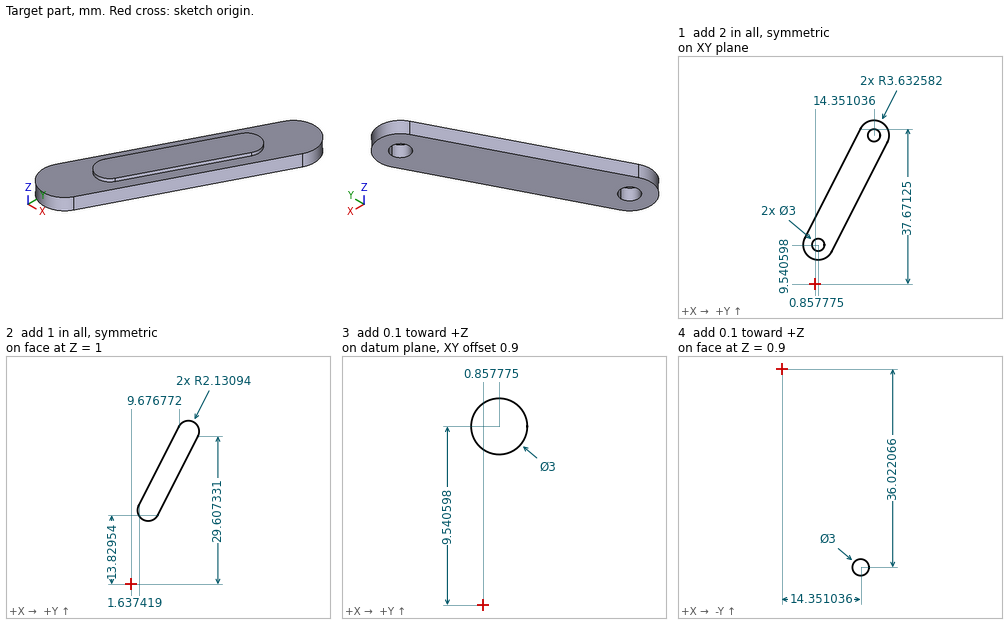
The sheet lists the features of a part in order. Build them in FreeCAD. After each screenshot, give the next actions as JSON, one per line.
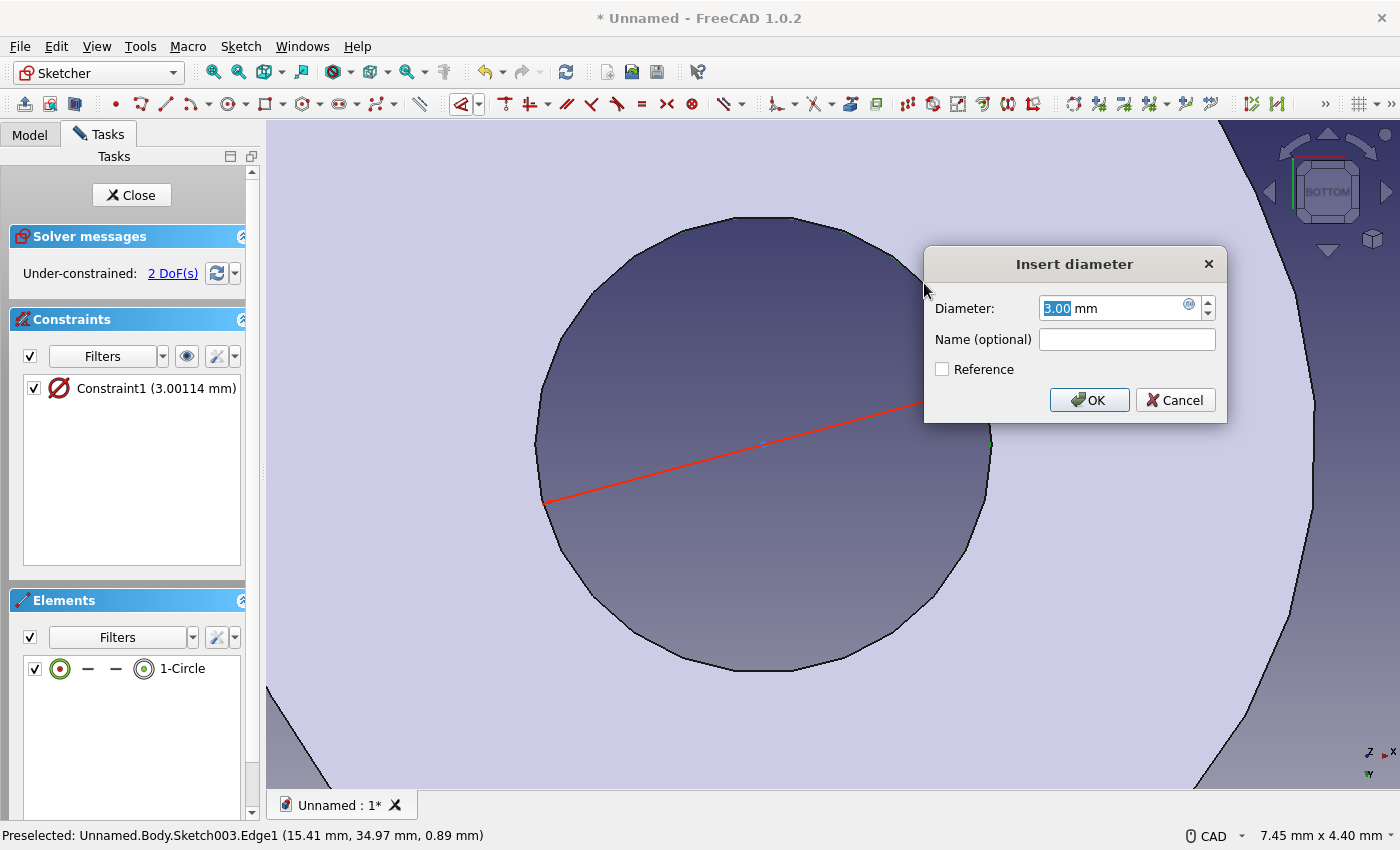
{"action": "type", "text": "3"}
{"action": "key", "text": "Return"}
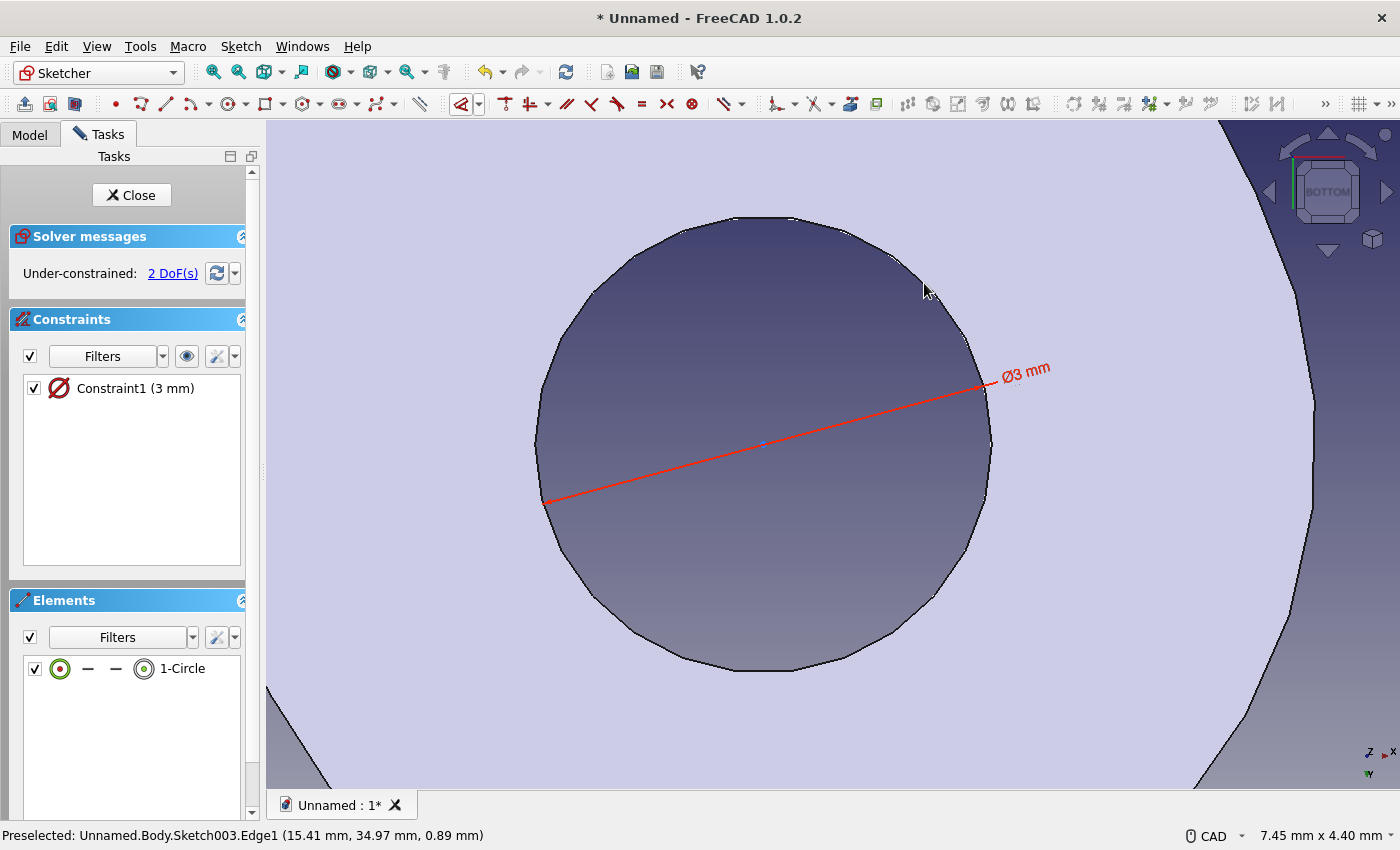
{"action": "left_click", "coordinate": [763, 445]}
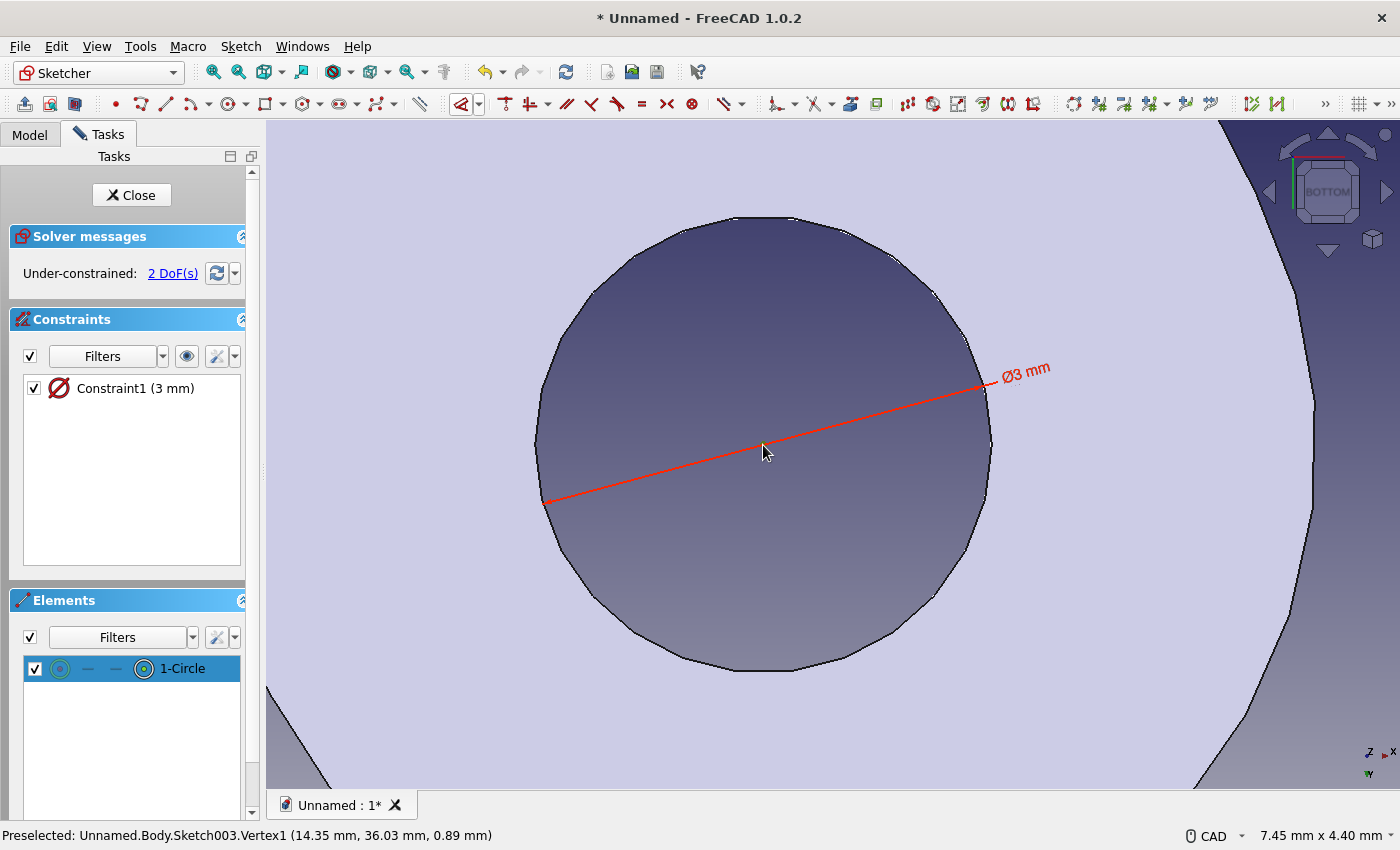
{"action": "key", "text": "l"}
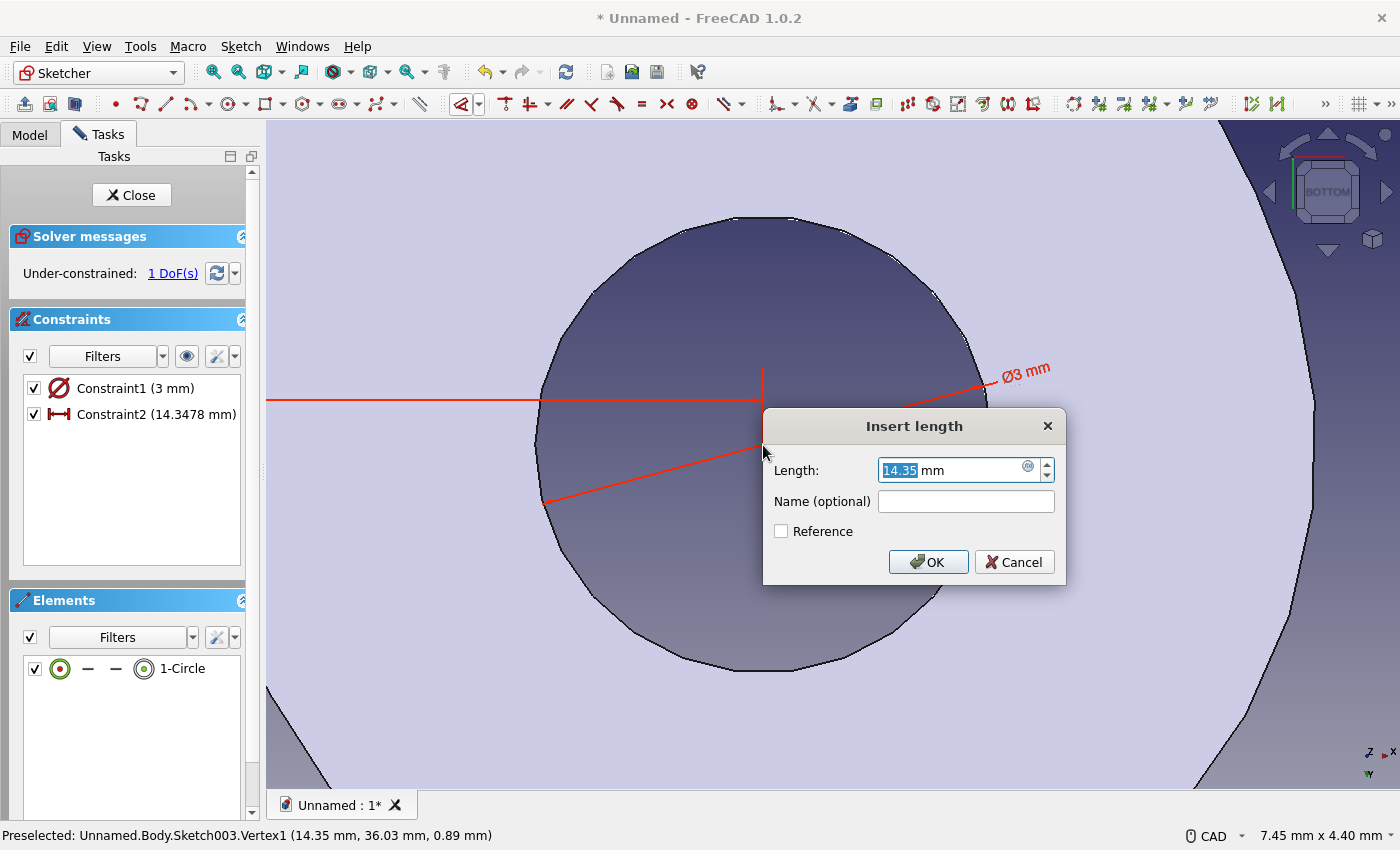
{"action": "type", "text": "14.351036"}
{"action": "key", "text": "Return"}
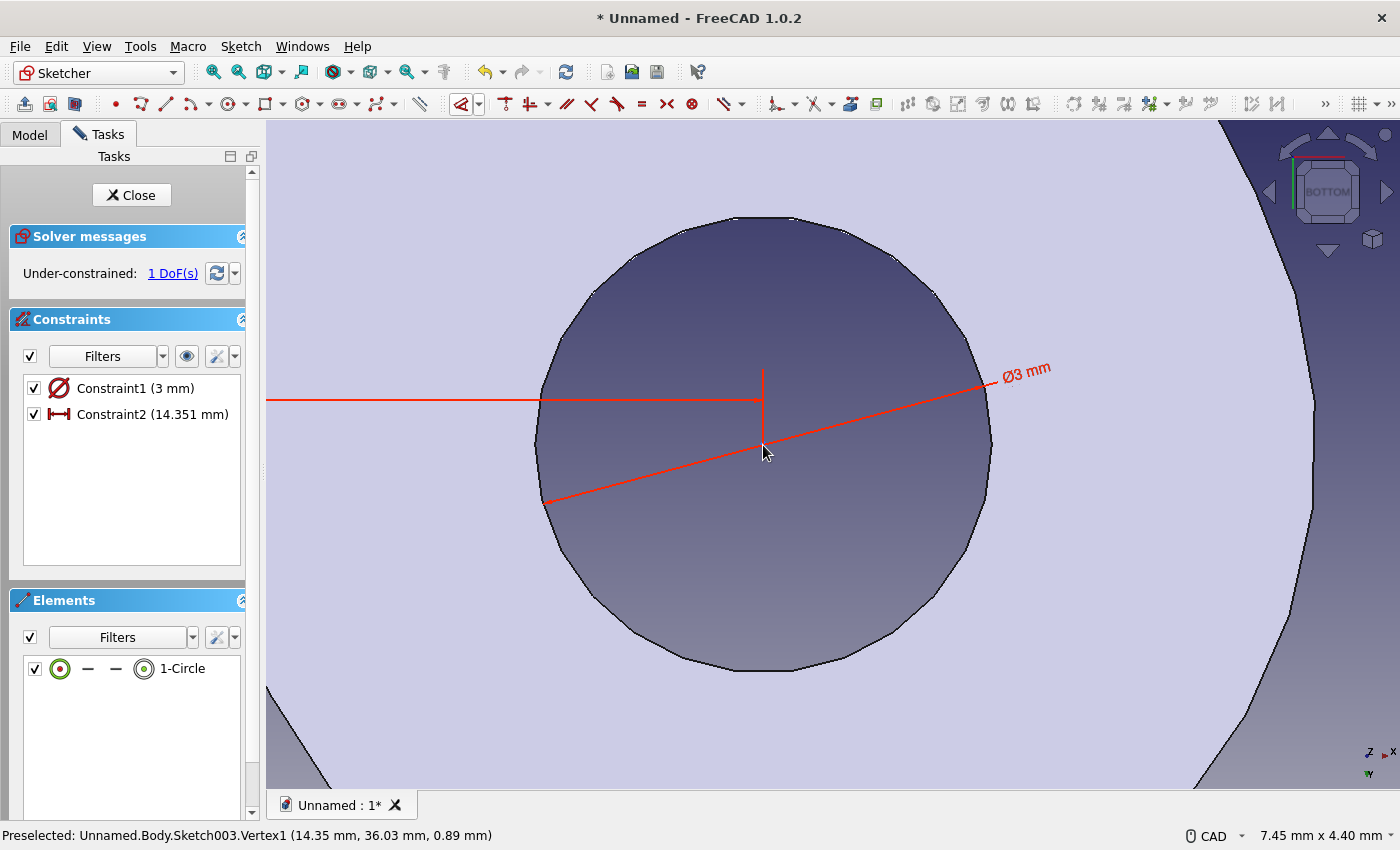
{"action": "left_click", "coordinate": [763, 445]}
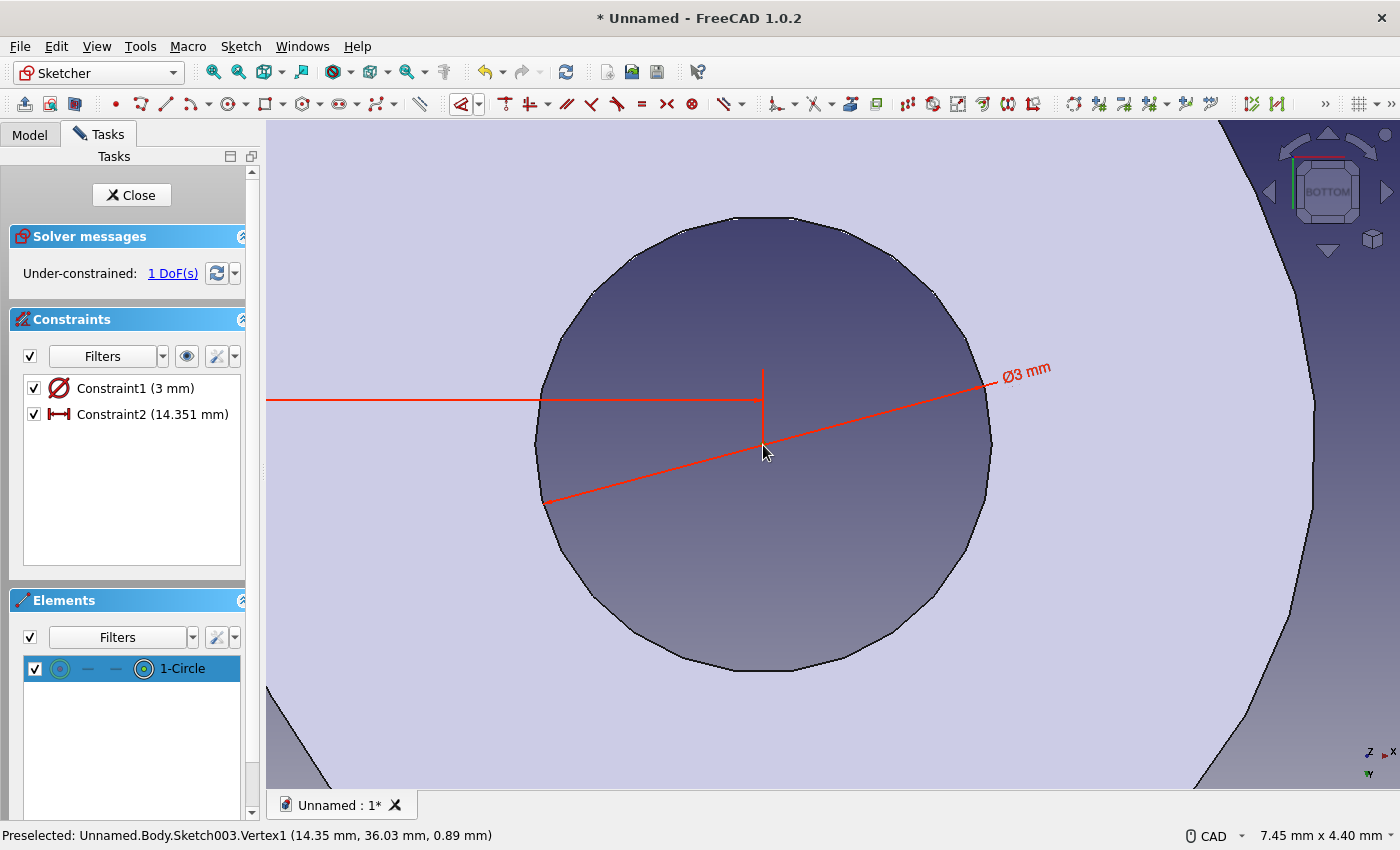
{"action": "key", "text": "i"}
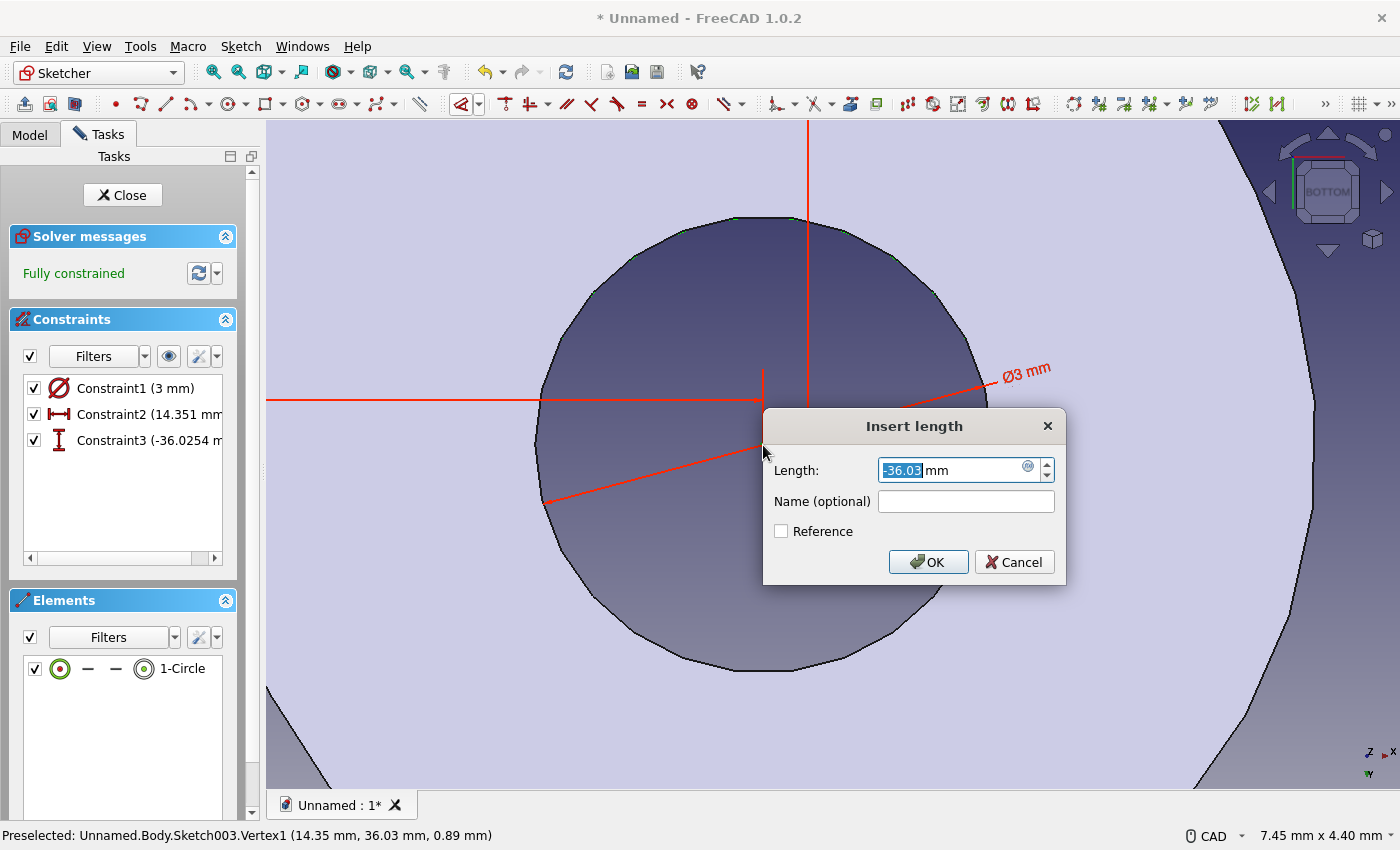
{"action": "type", "text": "-36.022066"}
{"action": "key", "text": "Return"}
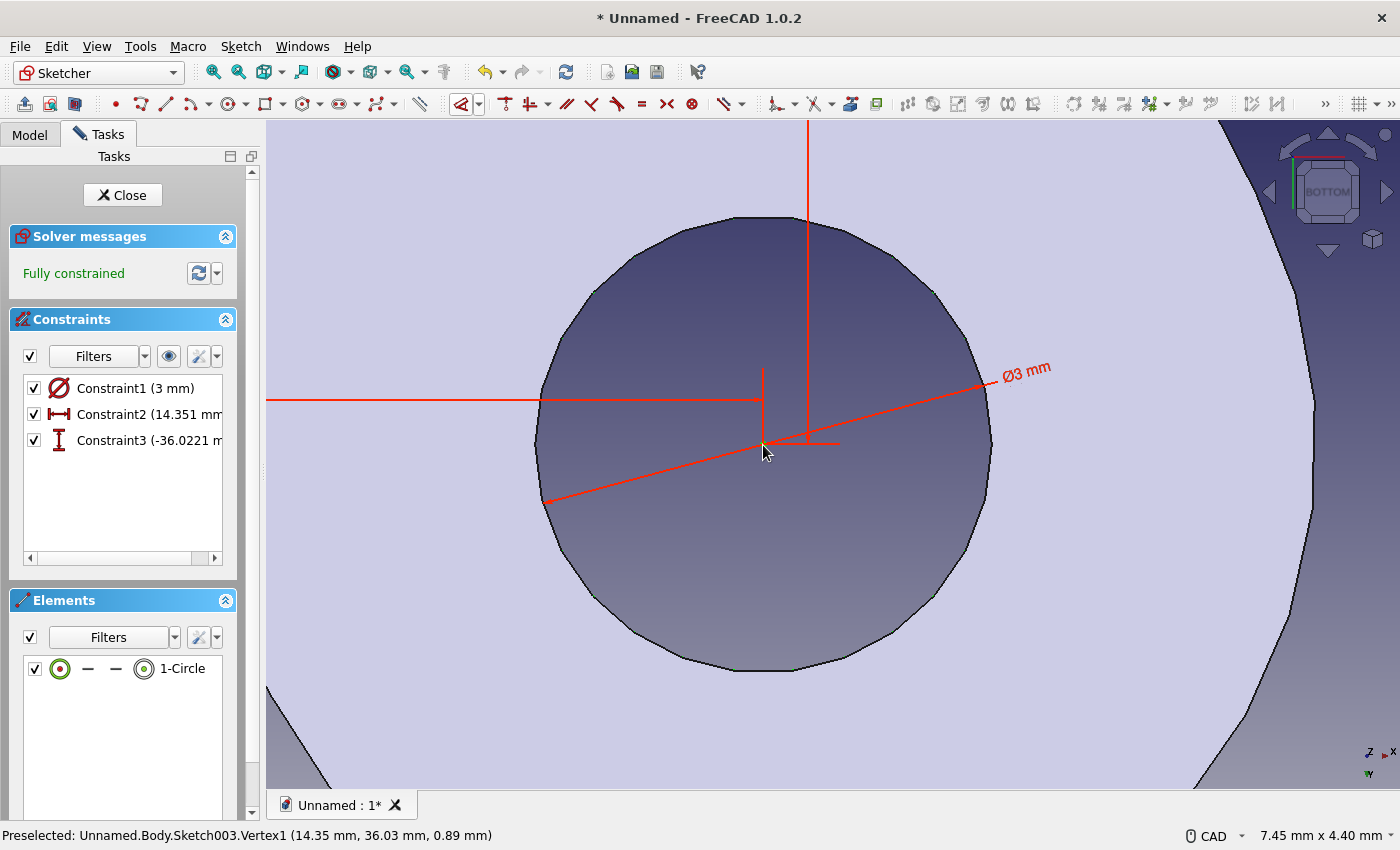
{"action": "left_click", "coordinate": [123, 195]}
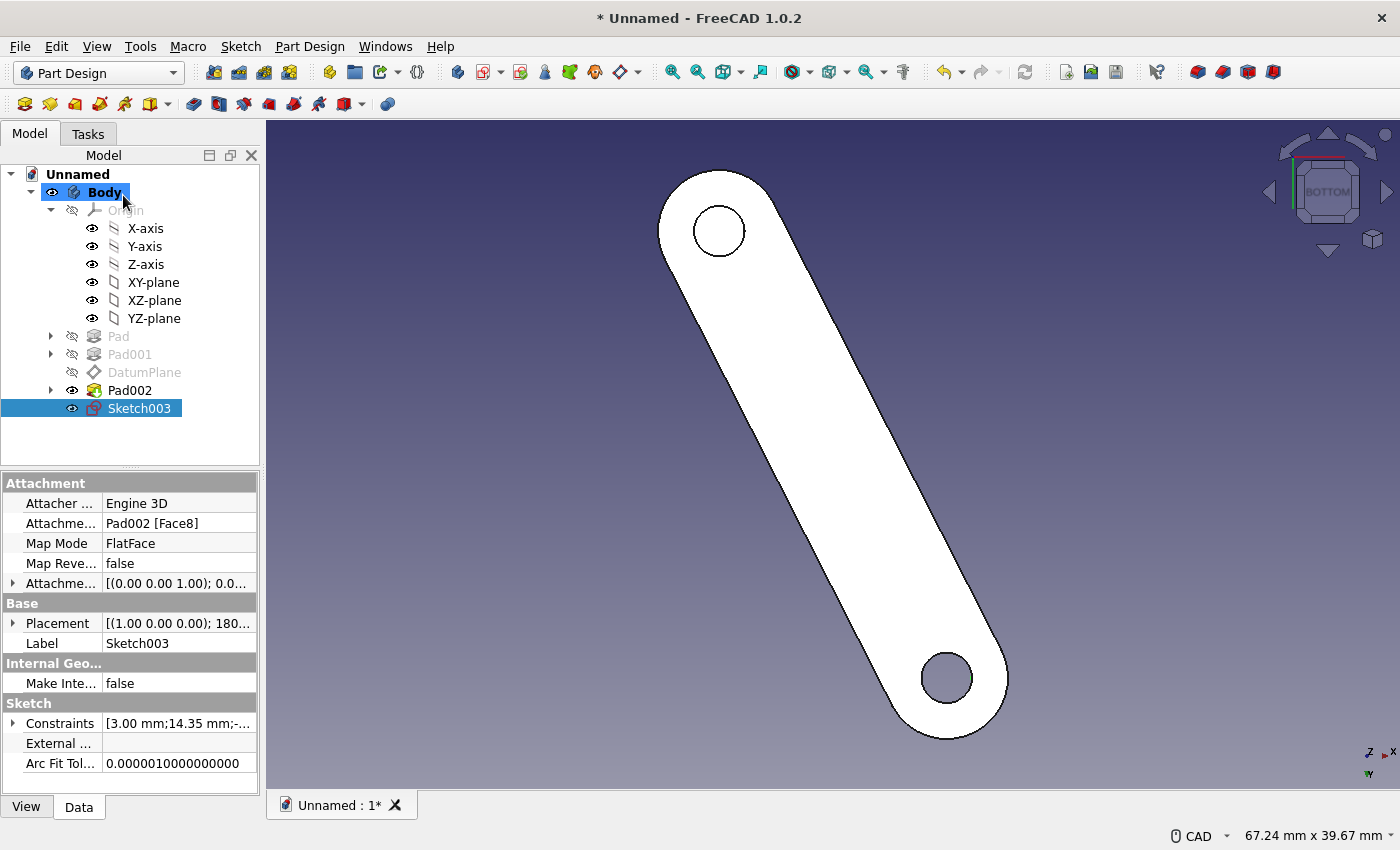
{"action": "left_click", "coordinate": [25, 104]}